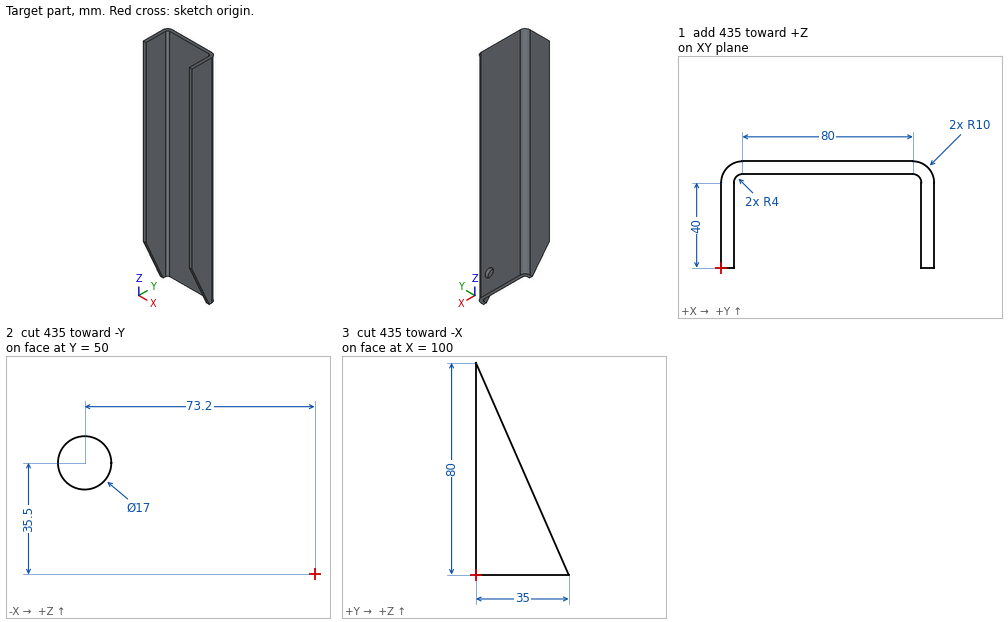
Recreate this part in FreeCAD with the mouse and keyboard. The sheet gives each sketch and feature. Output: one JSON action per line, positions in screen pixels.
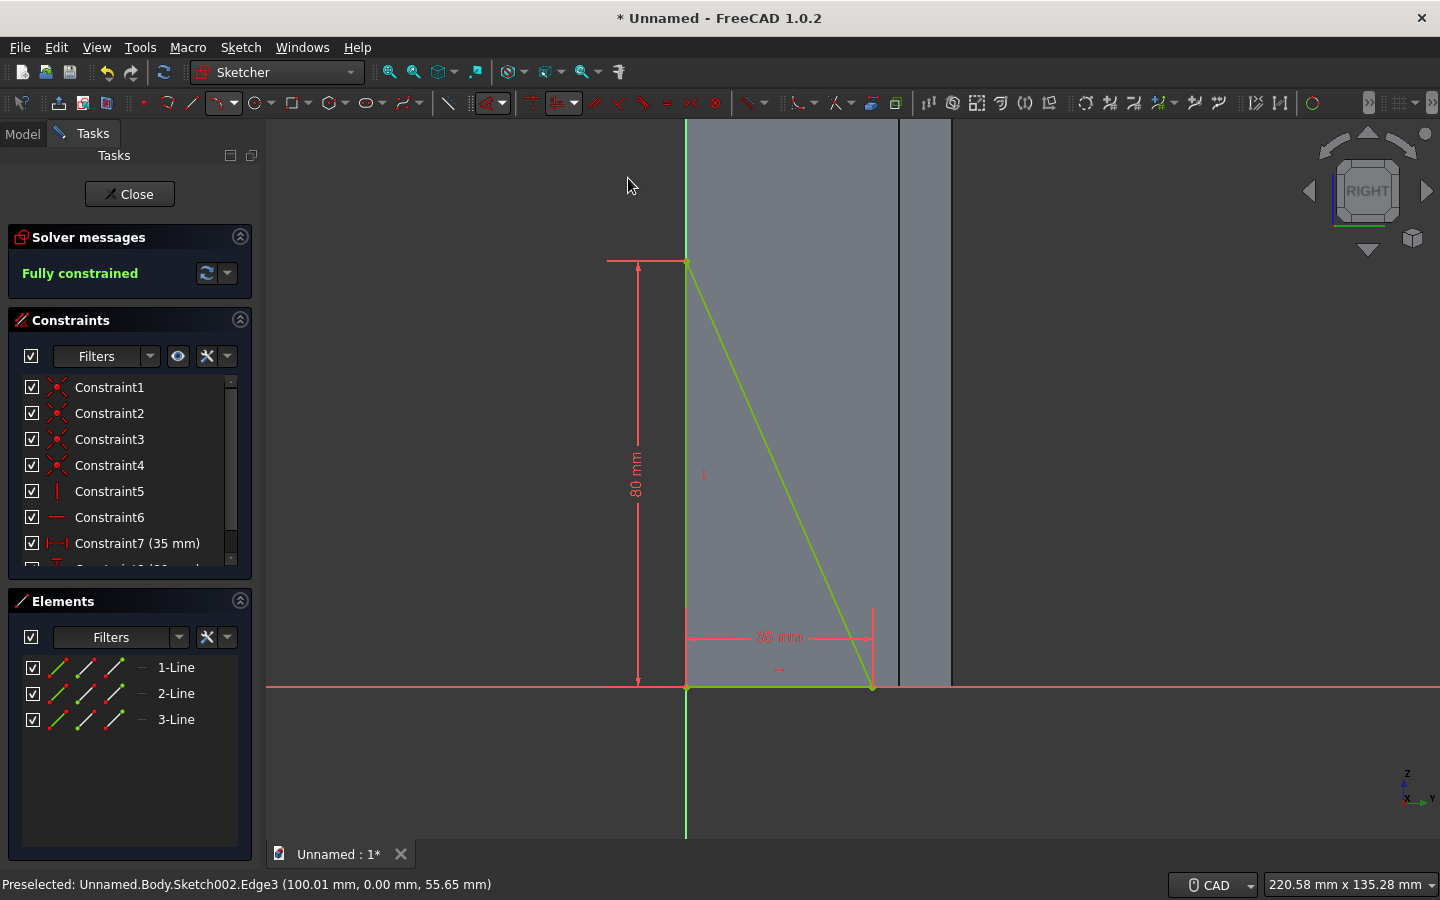
{"action": "left_click", "coordinate": [130, 194]}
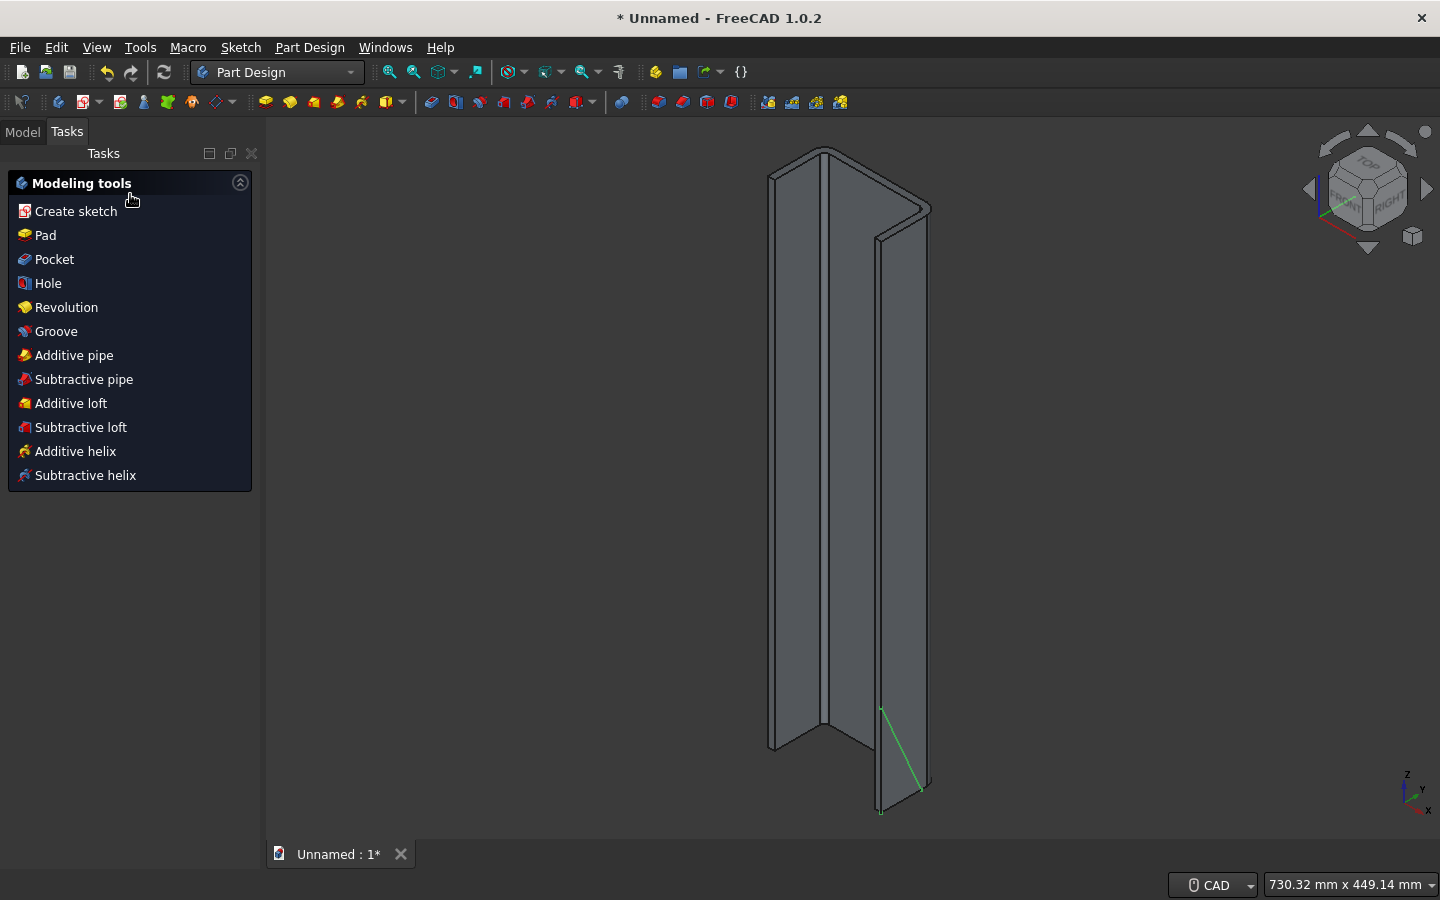
{"action": "left_click", "coordinate": [432, 102]}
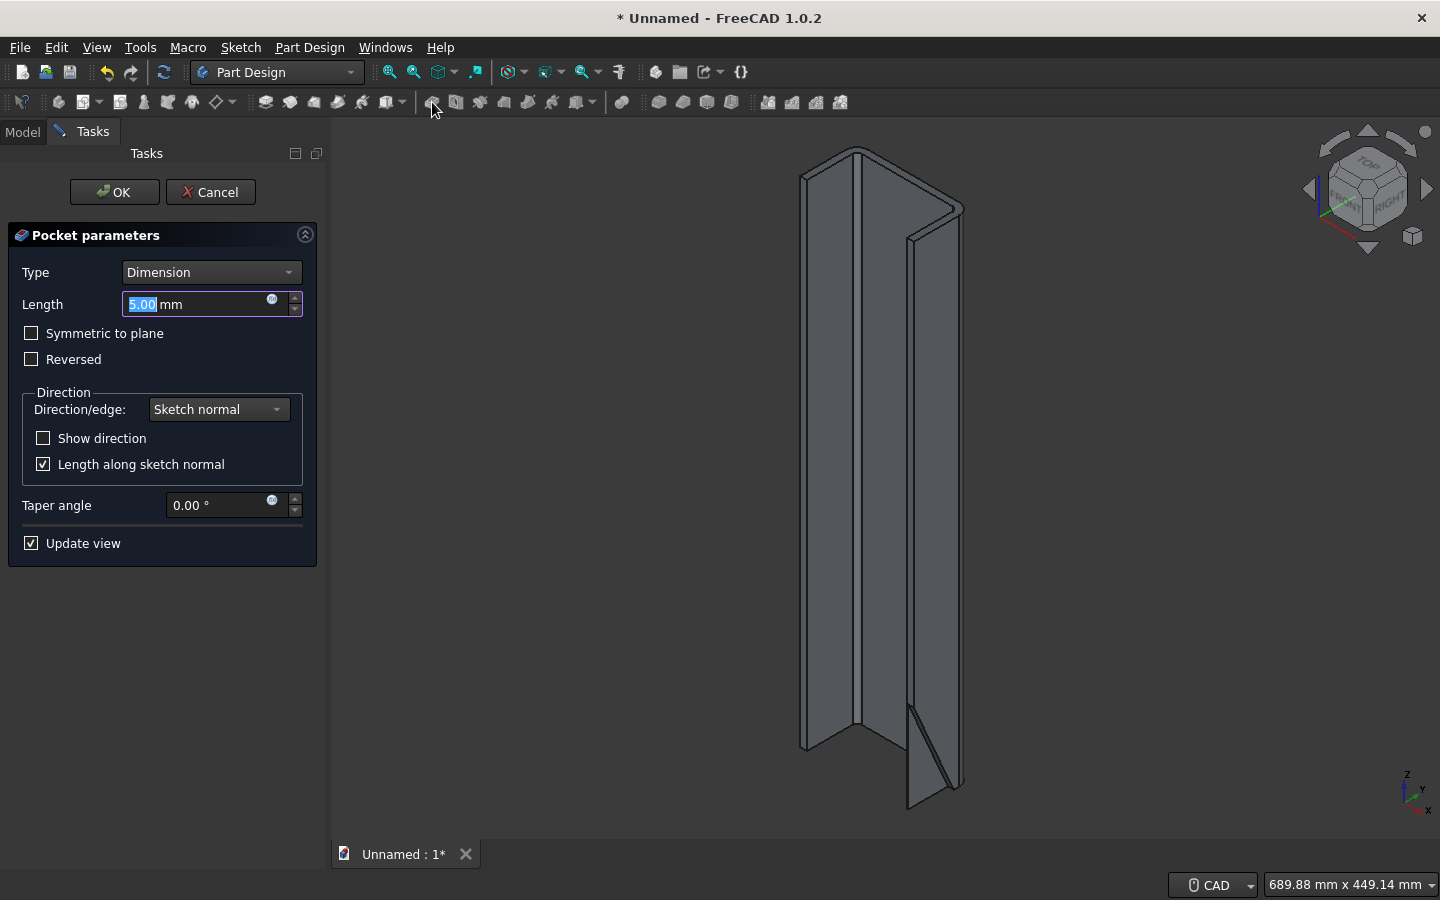
{"action": "type", "text": "435"}
{"action": "key", "text": "Tab"}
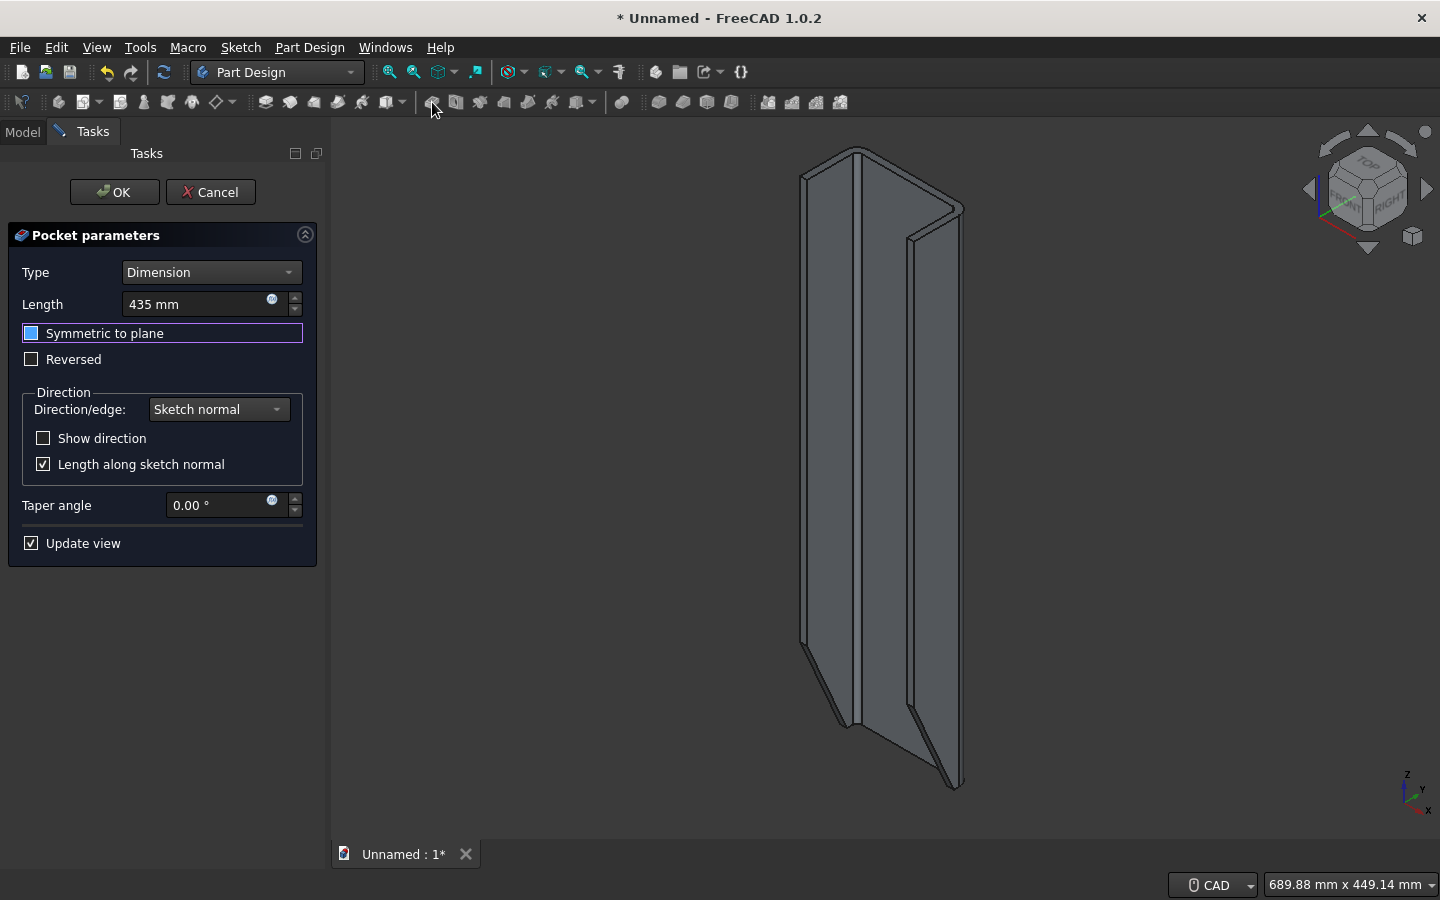
{"action": "left_click", "coordinate": [115, 192]}